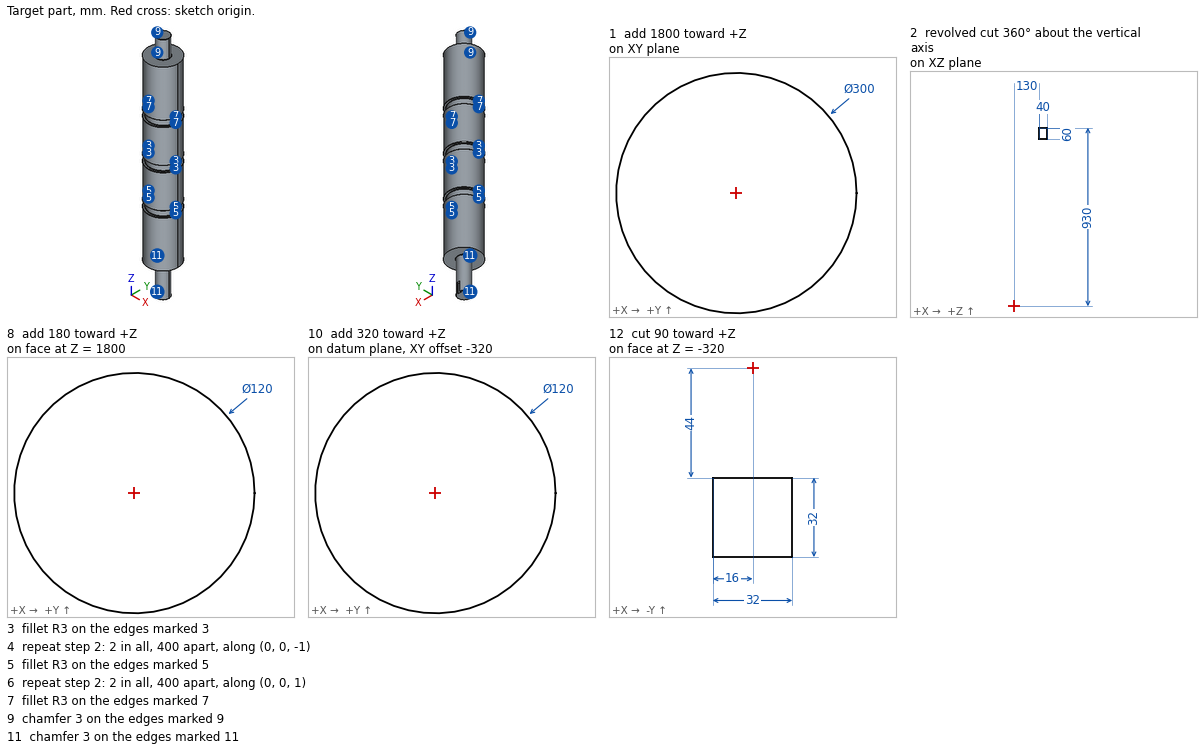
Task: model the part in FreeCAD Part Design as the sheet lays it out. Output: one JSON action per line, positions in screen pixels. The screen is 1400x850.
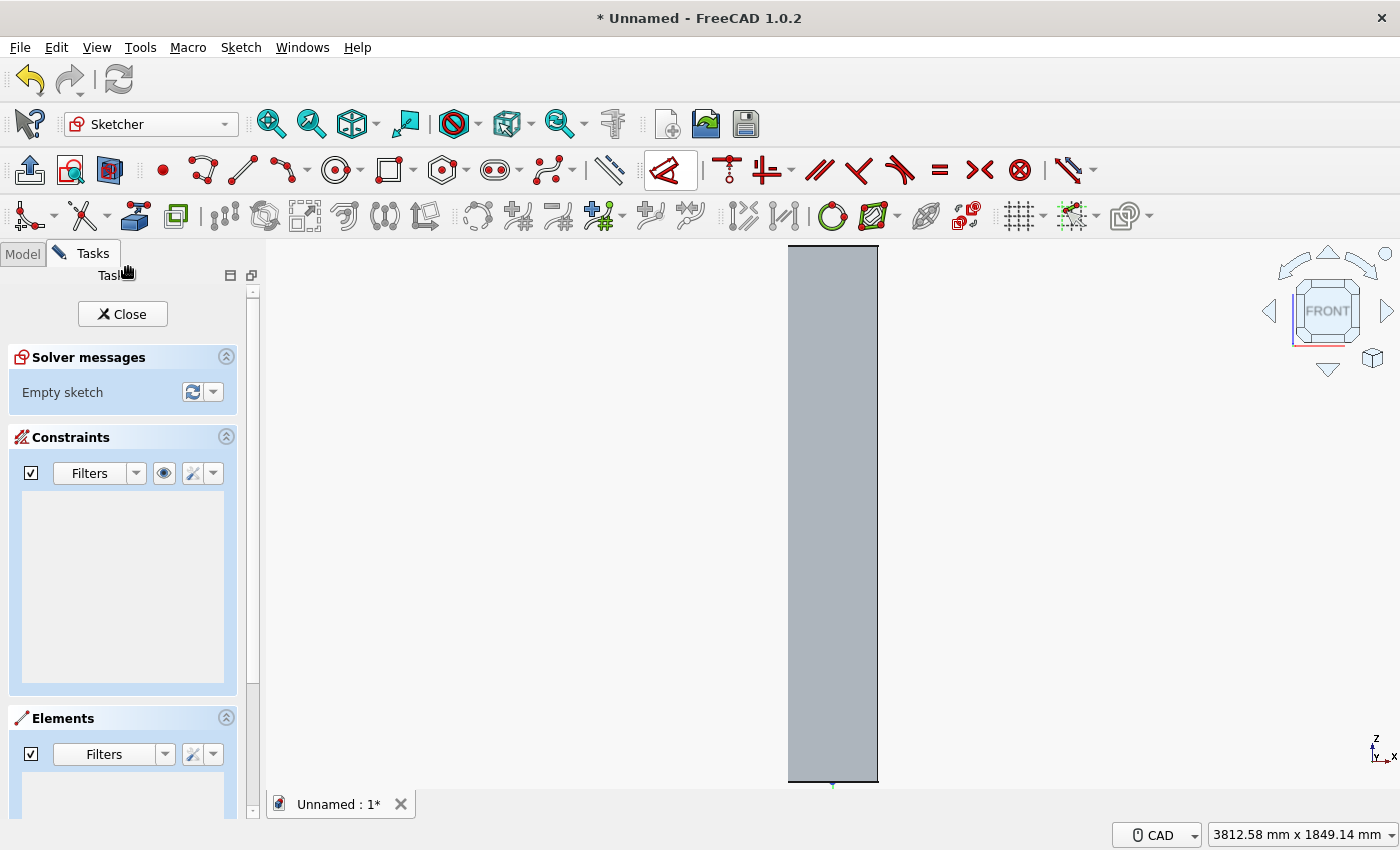
{"action": "left_click", "coordinate": [110, 170]}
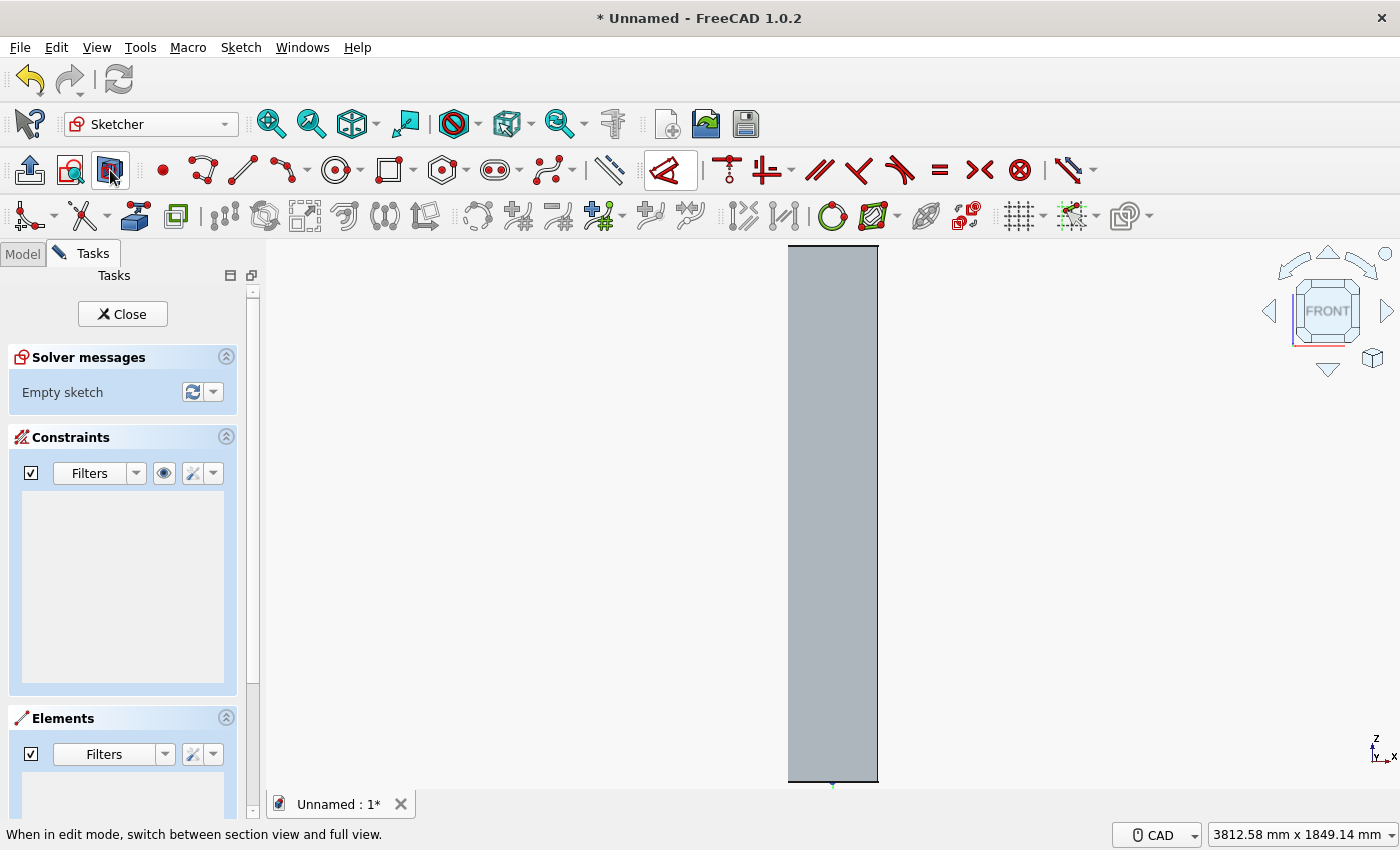
{"action": "scroll", "coordinate": [883, 514], "scroll_direction": "up", "scroll_amount": 15}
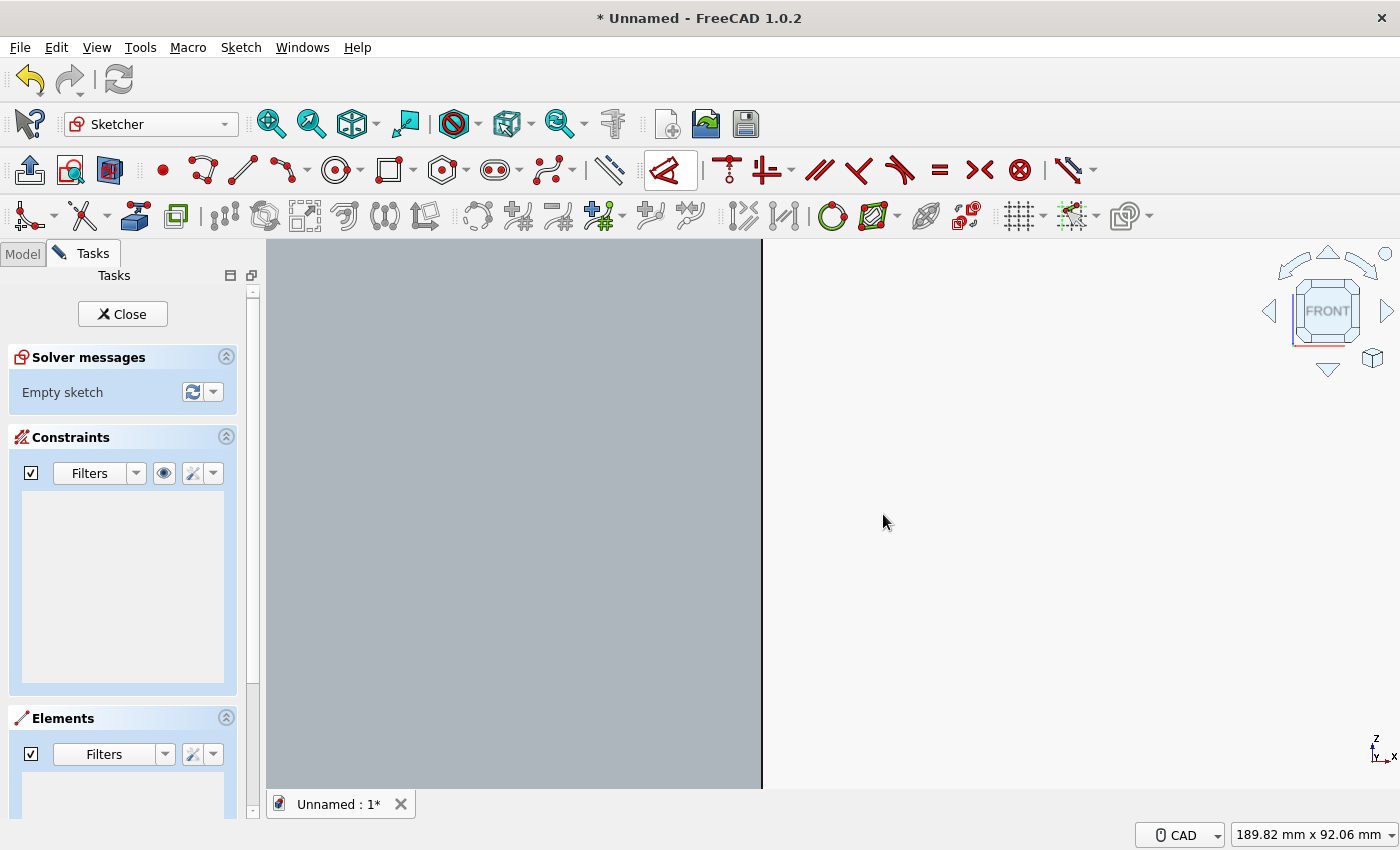
{"action": "left_click", "coordinate": [390, 170]}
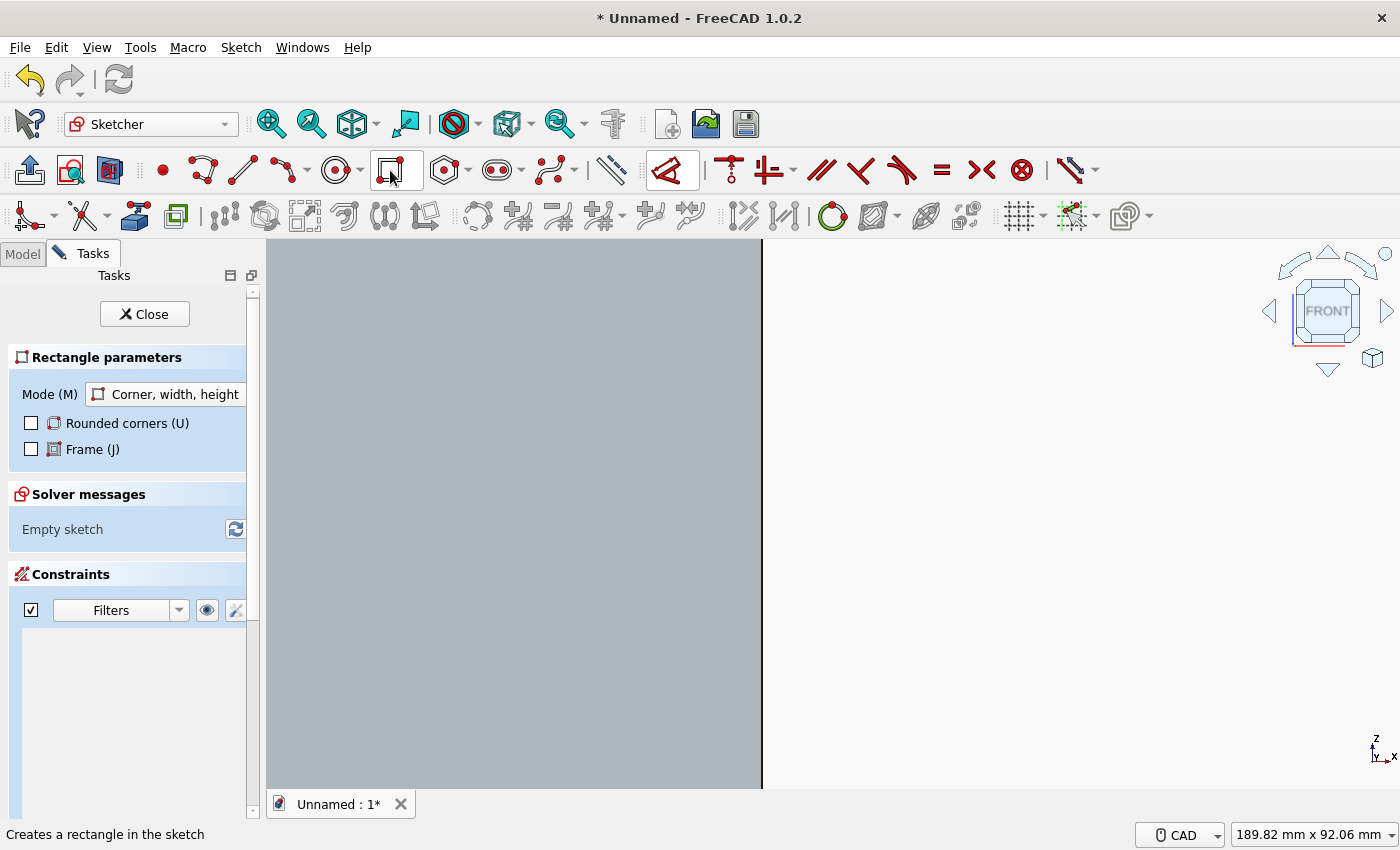
{"action": "left_click", "coordinate": [643, 325]}
{"action": "mouse_move", "coordinate": [882, 684]}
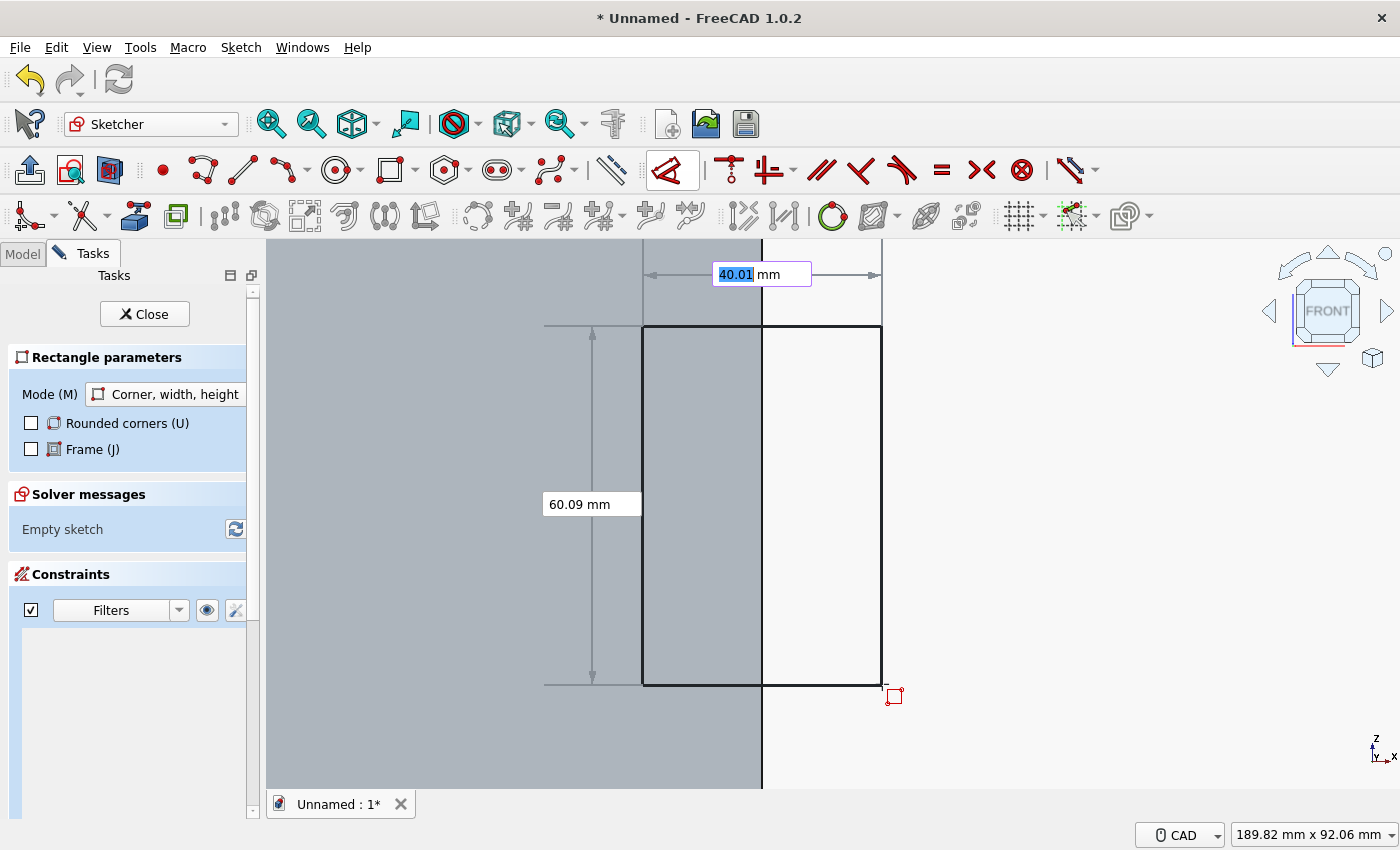
{"action": "type", "text": "40"}
{"action": "key", "text": "Tab"}
{"action": "type", "text": "60"}
{"action": "key", "text": "Return"}
{"action": "key", "text": "Escape"}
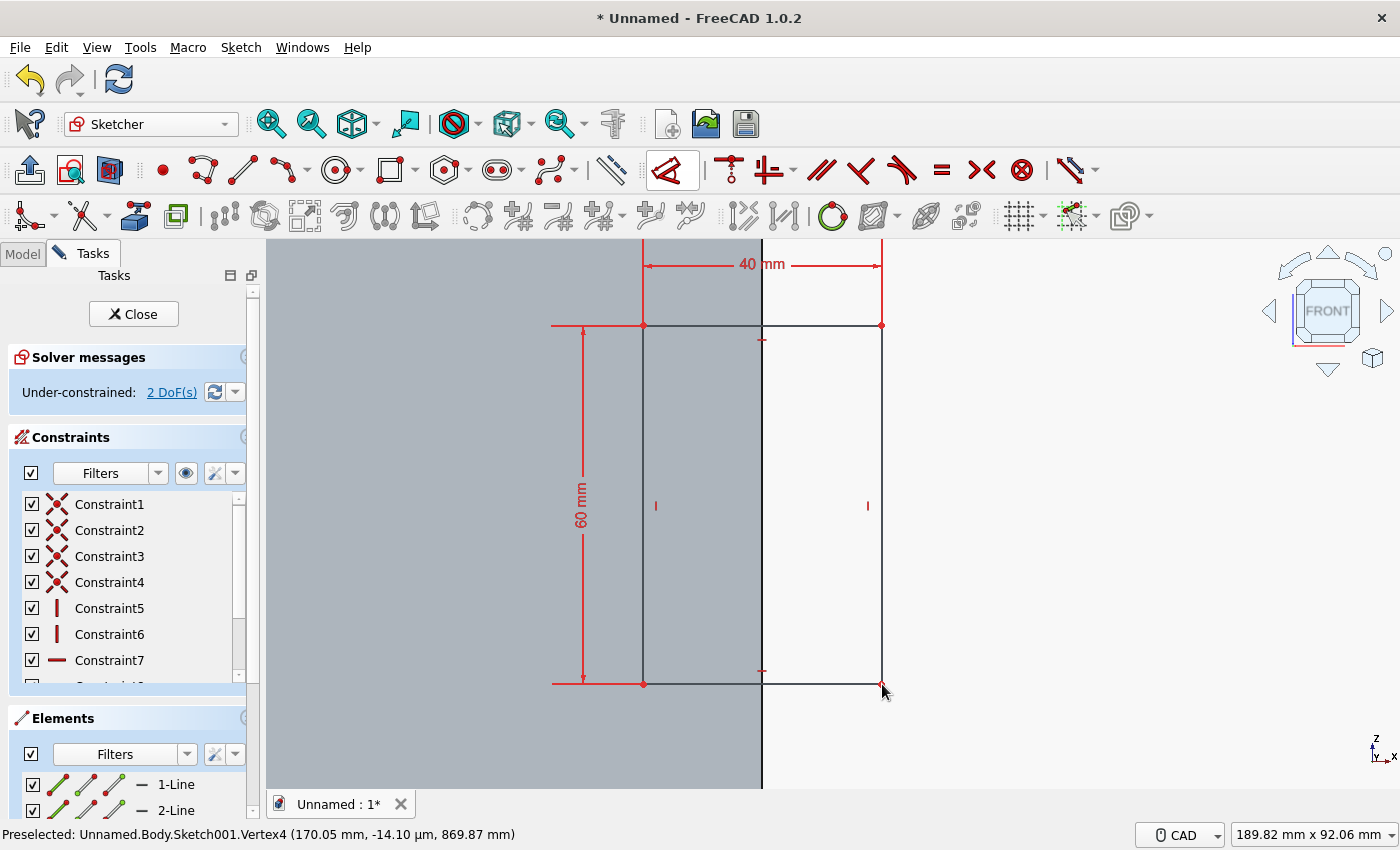
{"action": "left_click", "coordinate": [666, 170]}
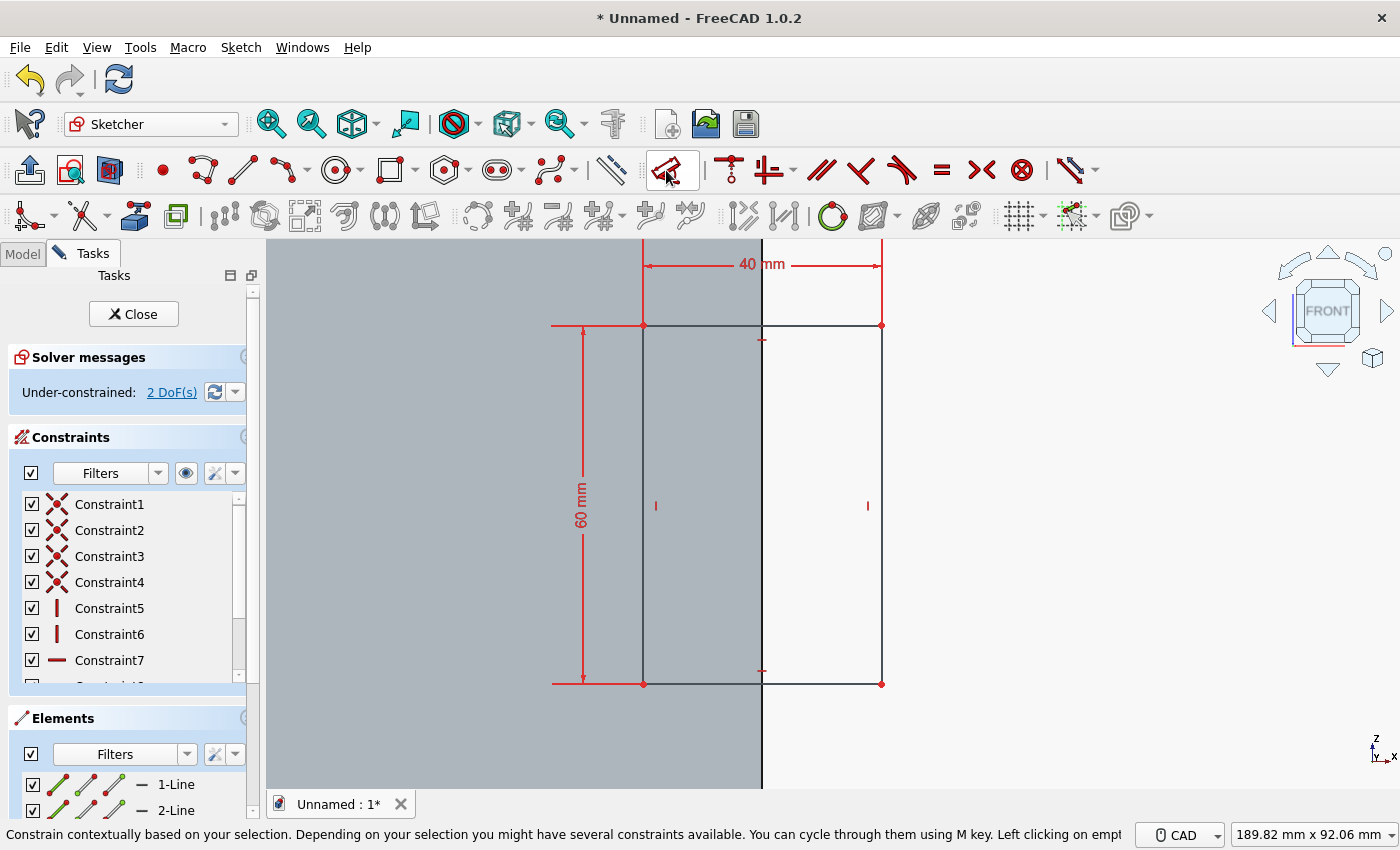
{"action": "left_click", "coordinate": [643, 326]}
{"action": "left_click", "coordinate": [468, 292]}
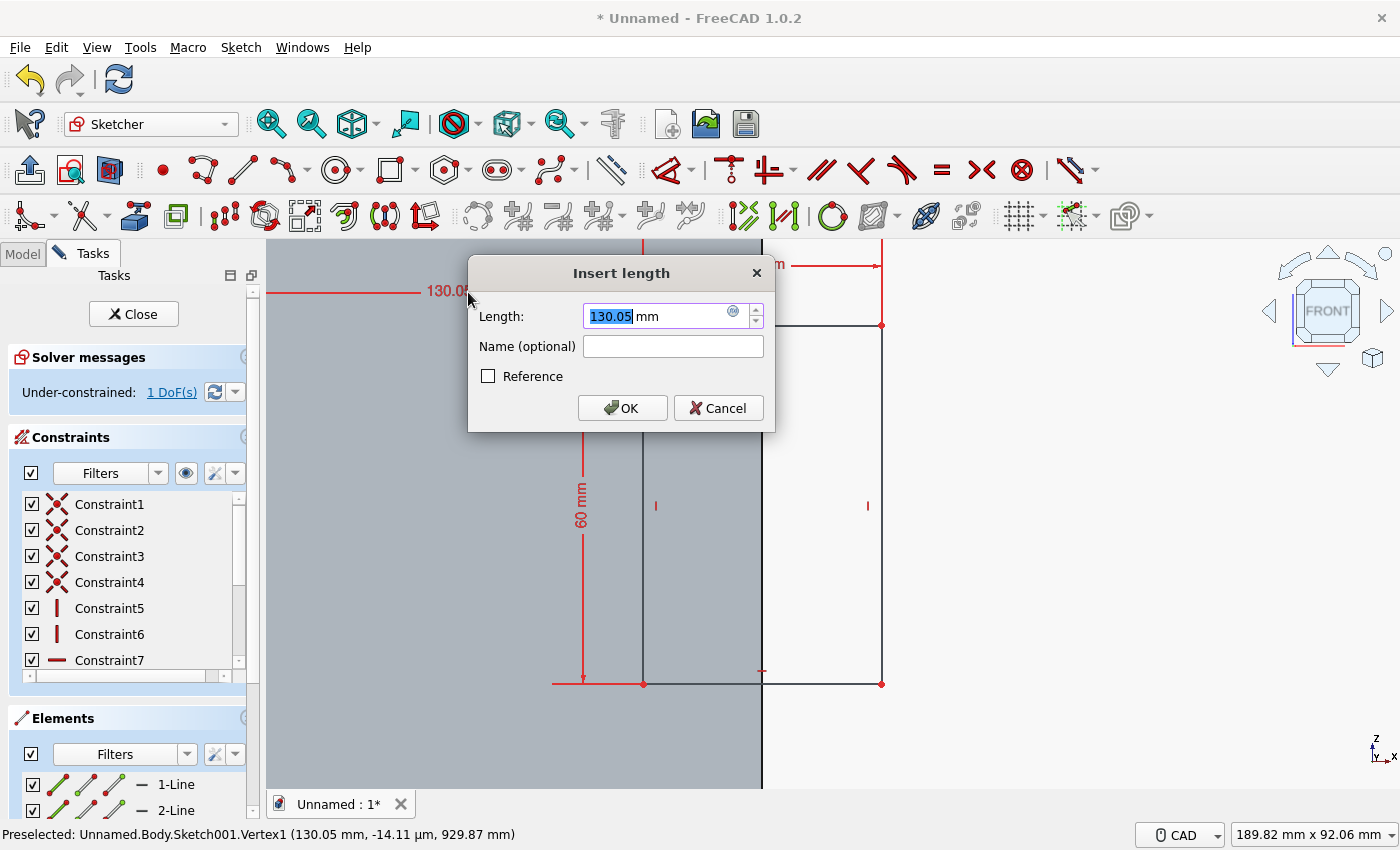
{"action": "type", "text": "130"}
{"action": "key", "text": "Return"}